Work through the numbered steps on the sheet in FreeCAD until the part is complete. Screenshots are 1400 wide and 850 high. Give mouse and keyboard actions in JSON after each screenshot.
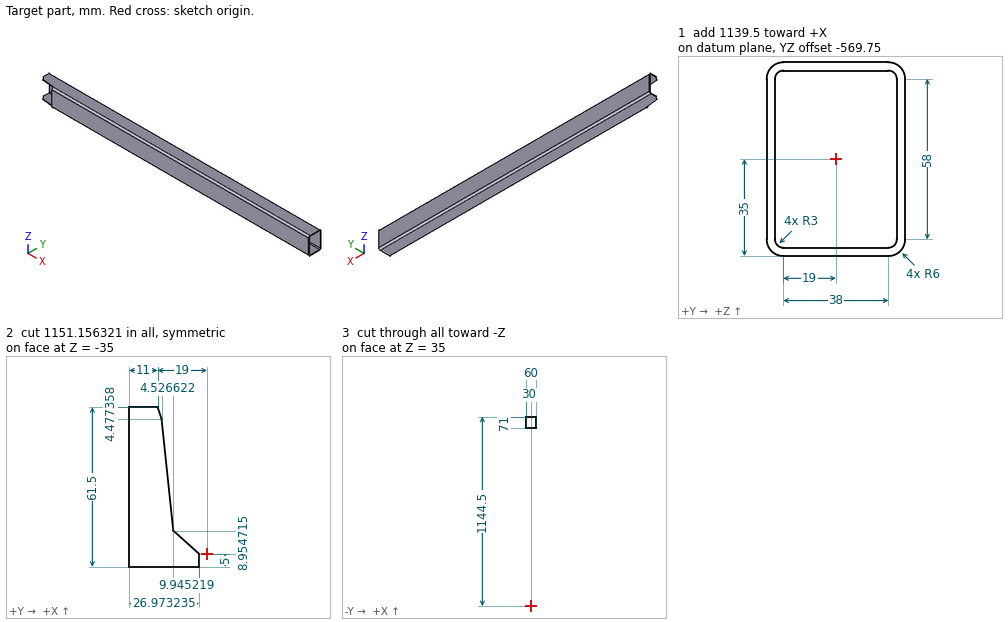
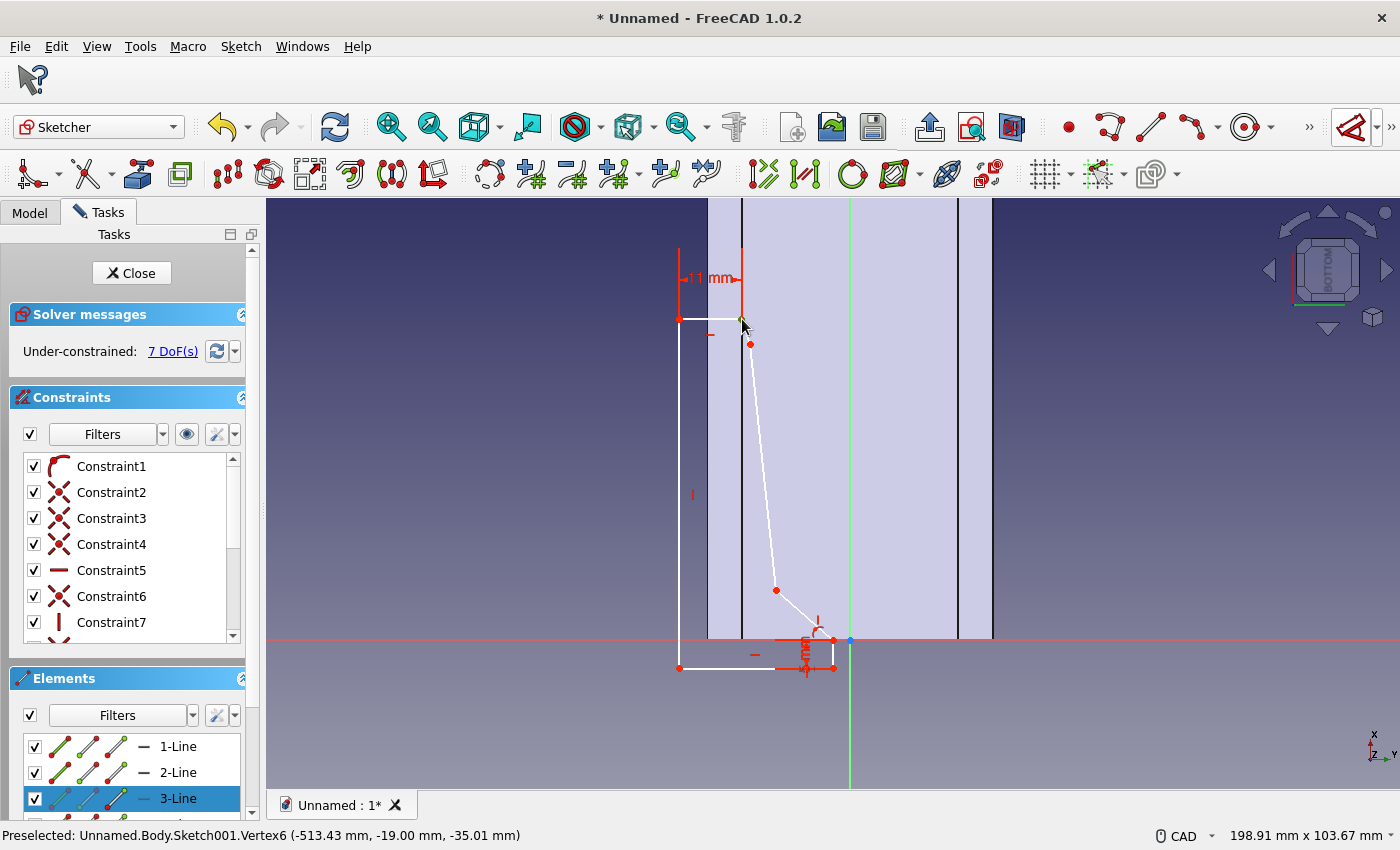
{"action": "left_click", "coordinate": [1376, 128]}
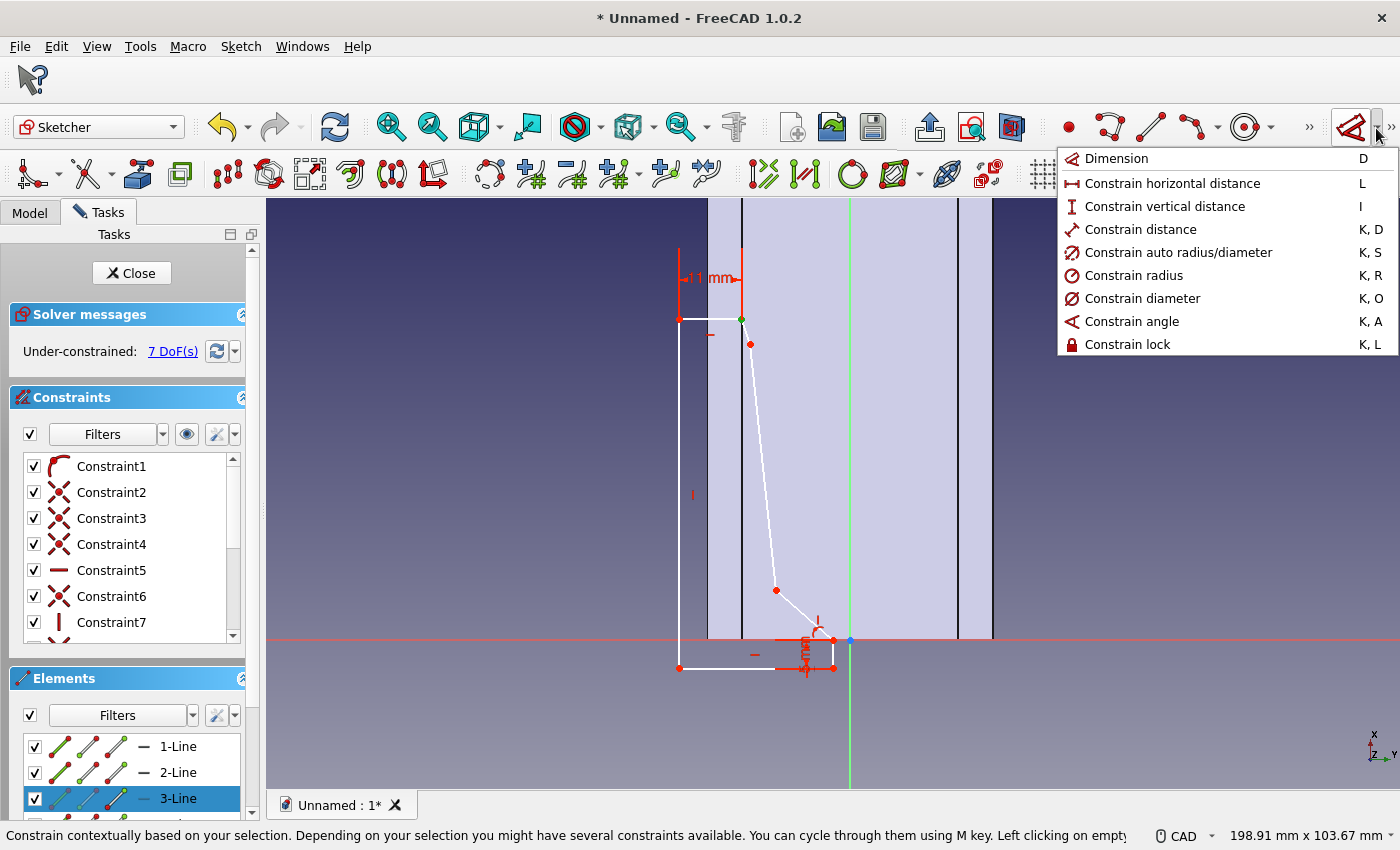
{"action": "left_click", "coordinate": [1228, 184]}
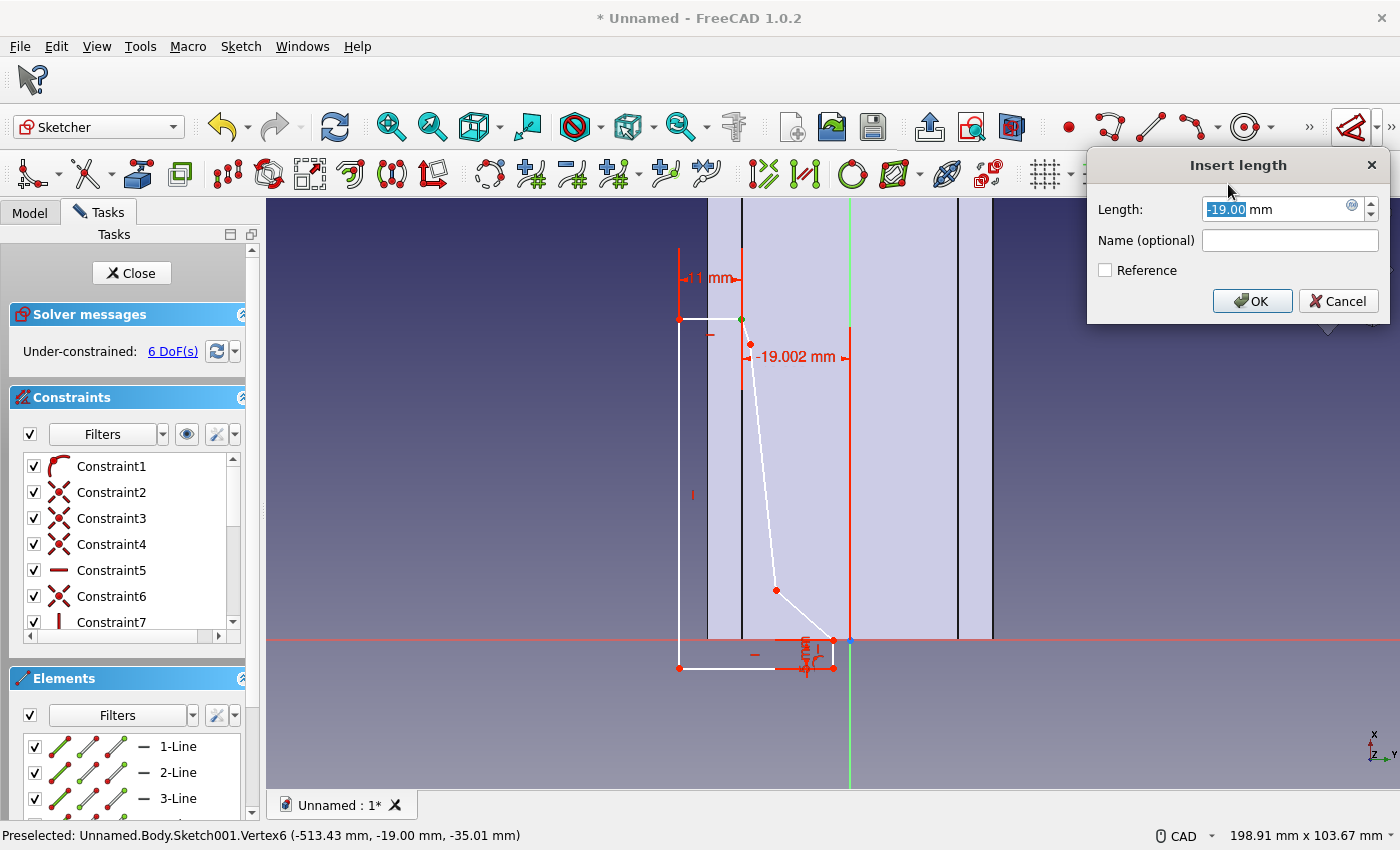
{"action": "type", "text": "-19"}
{"action": "key", "text": "Return"}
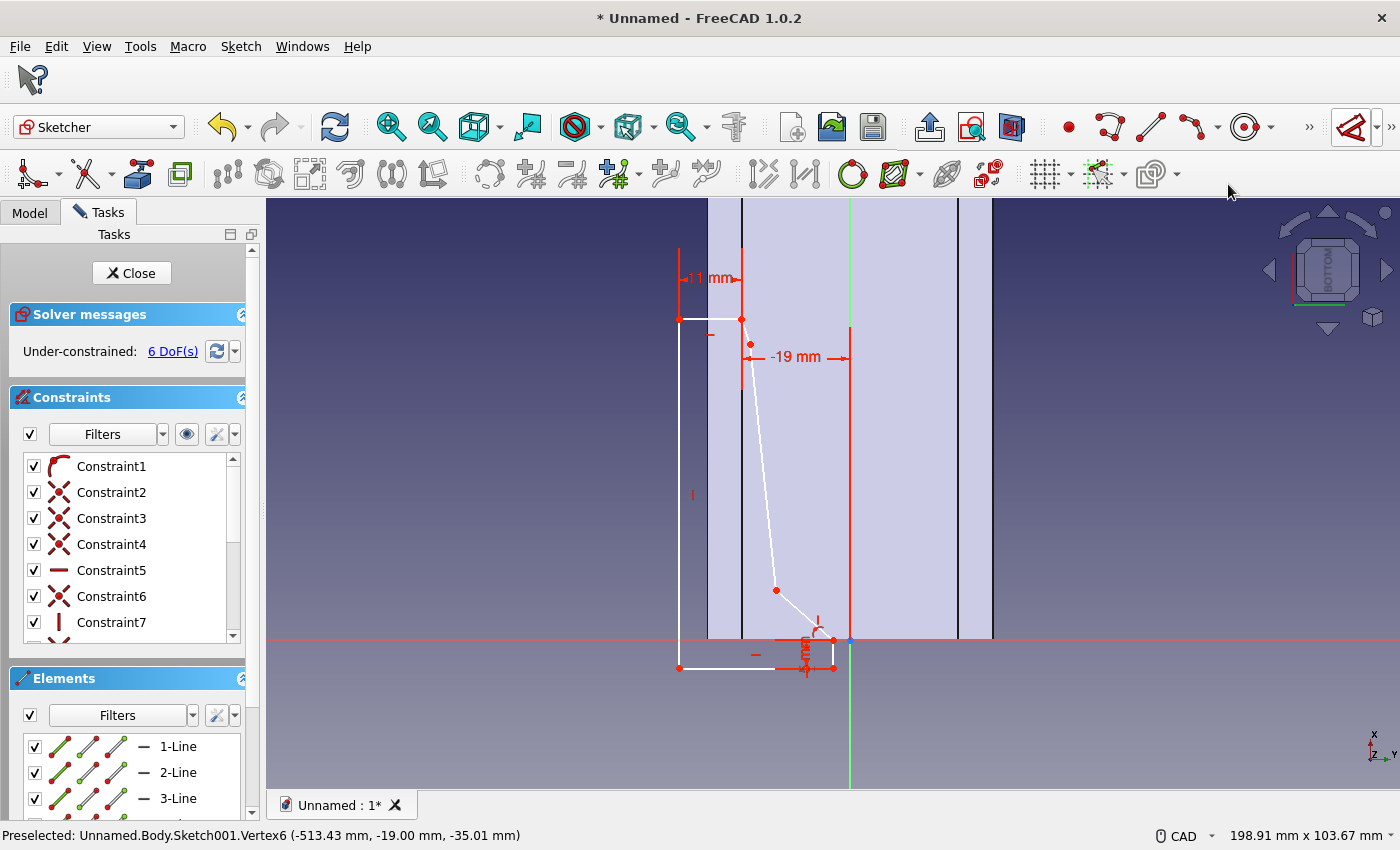
{"action": "left_click", "coordinate": [679, 424]}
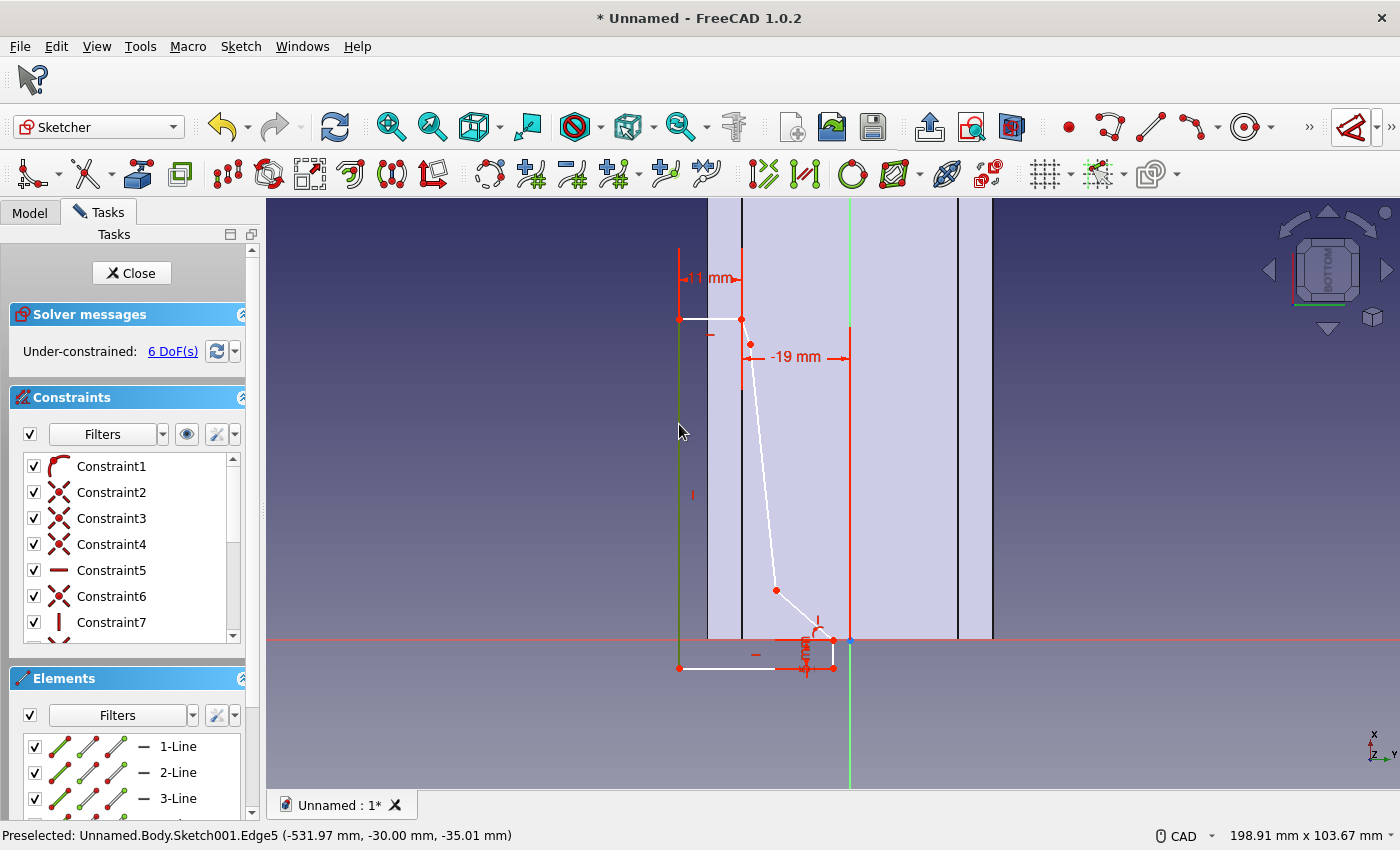
{"action": "key", "text": "i"}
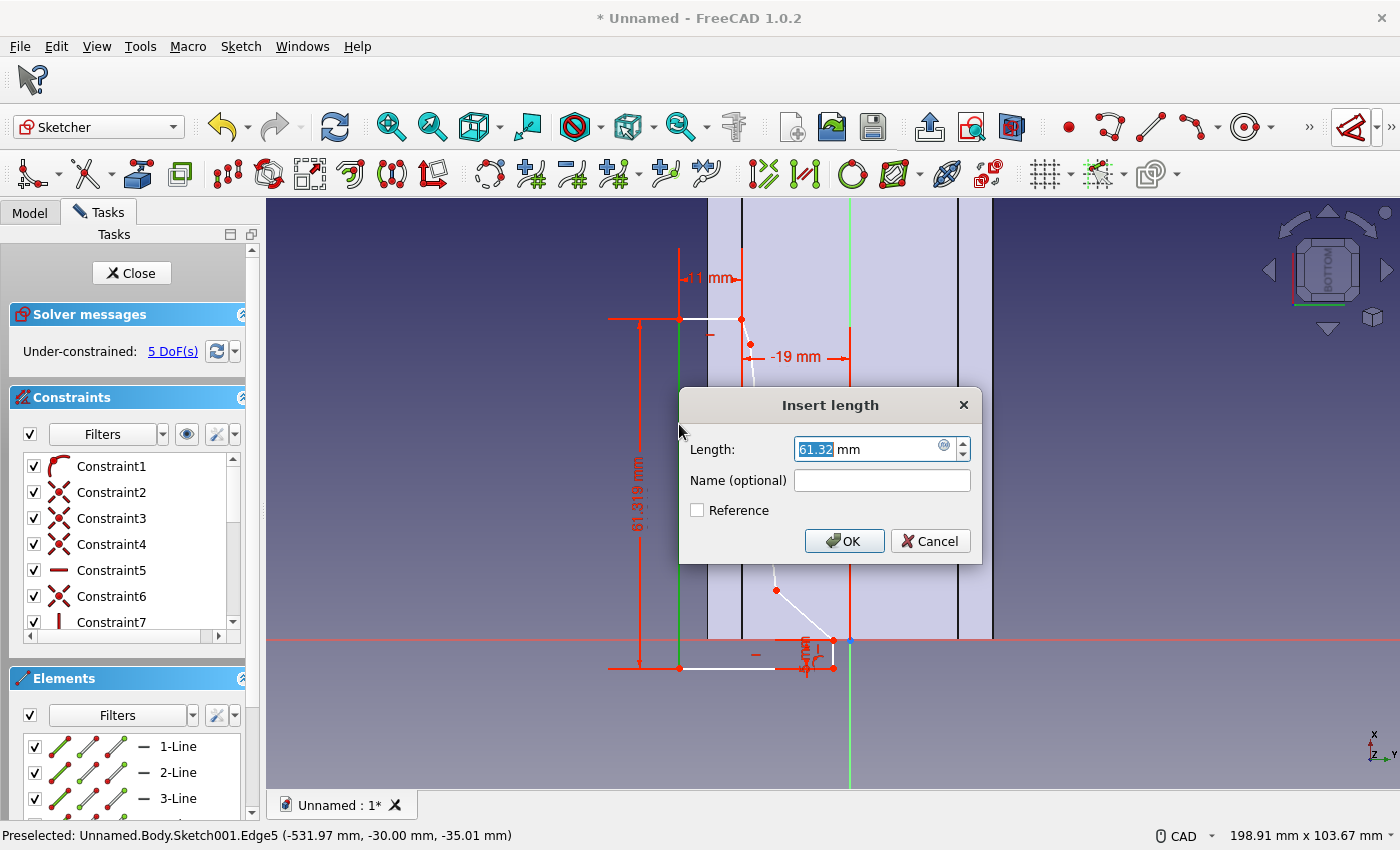
{"action": "type", "text": "61.5"}
{"action": "key", "text": "Return"}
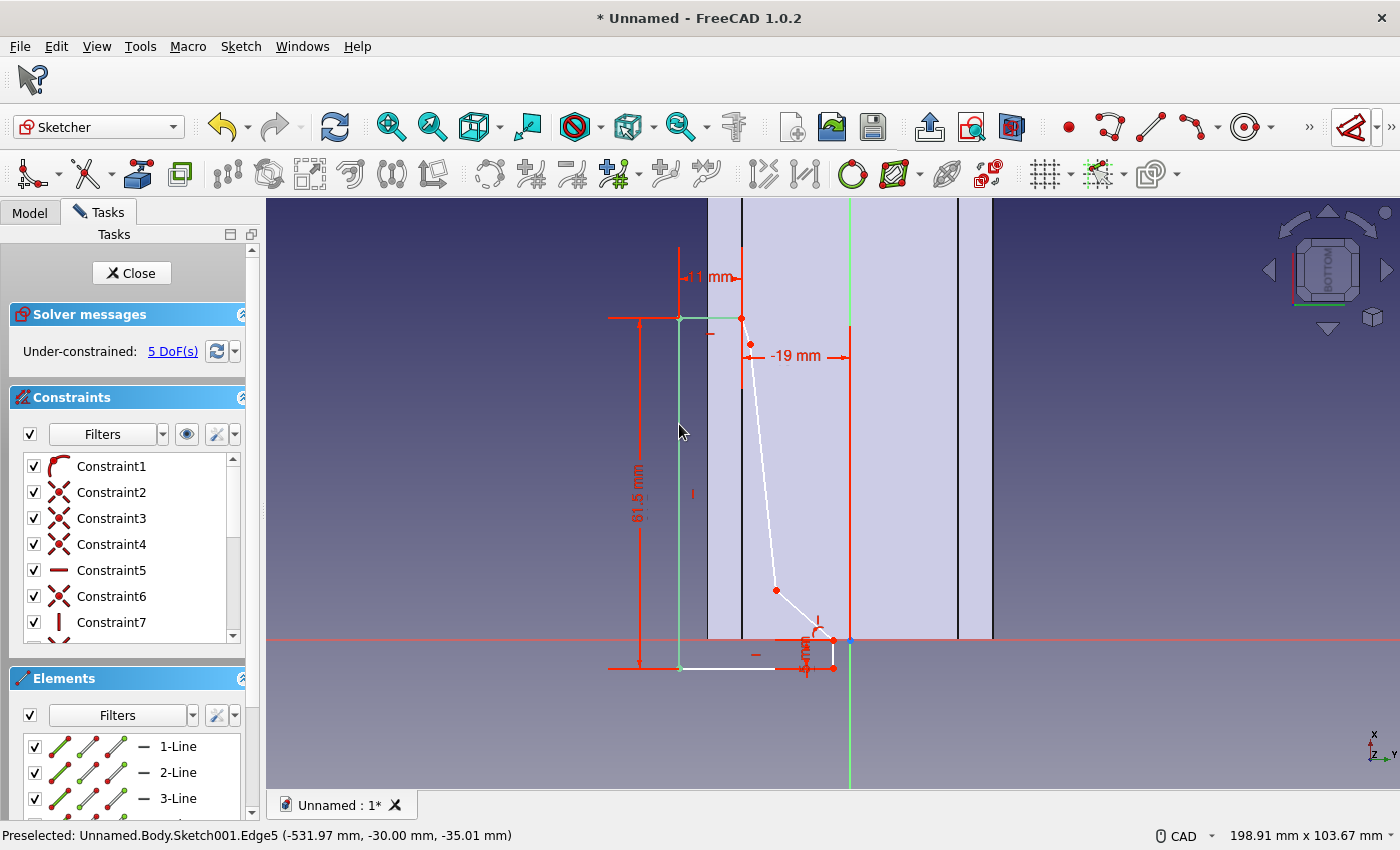
{"action": "left_click", "coordinate": [725, 669]}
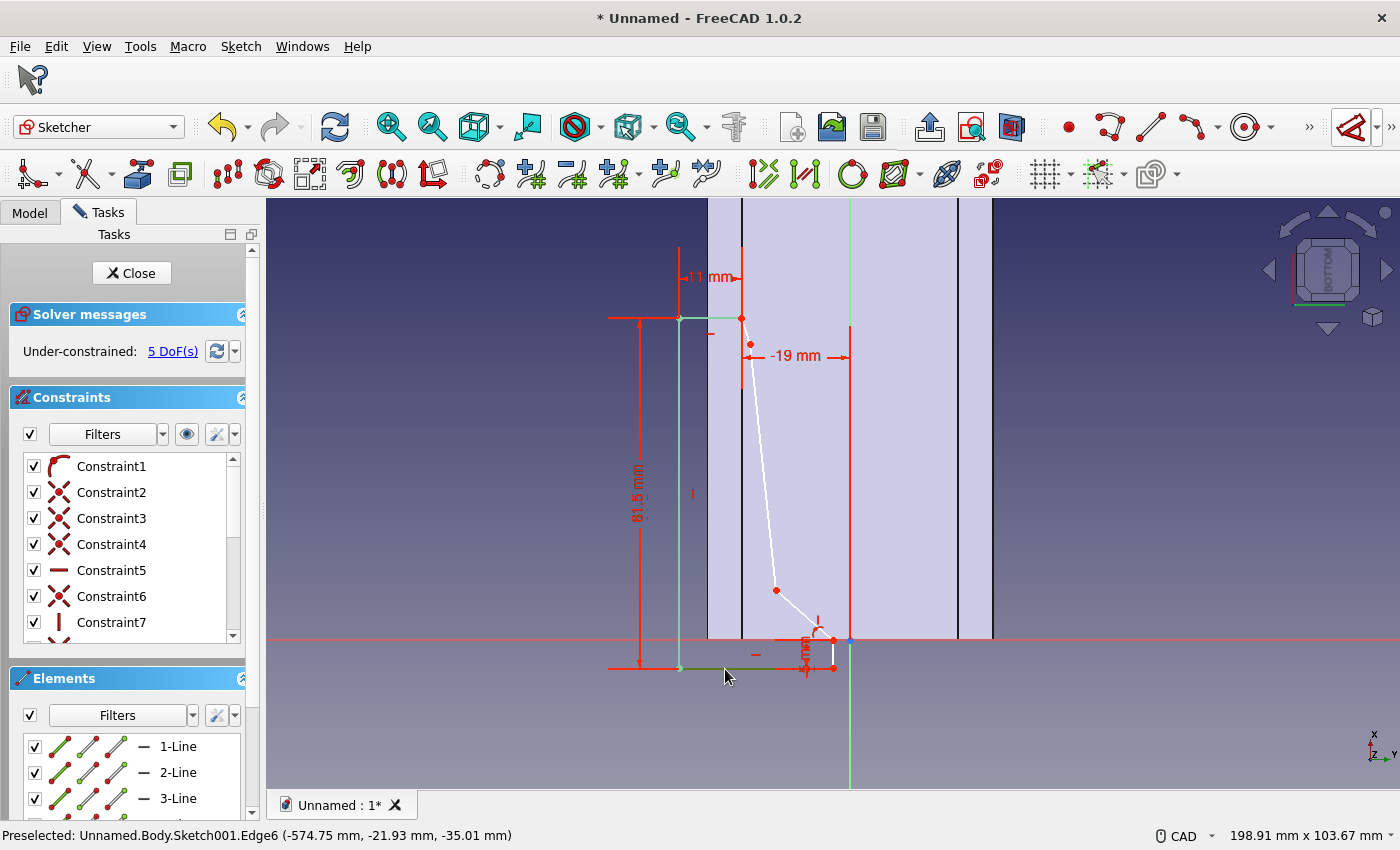
{"action": "key", "text": "l"}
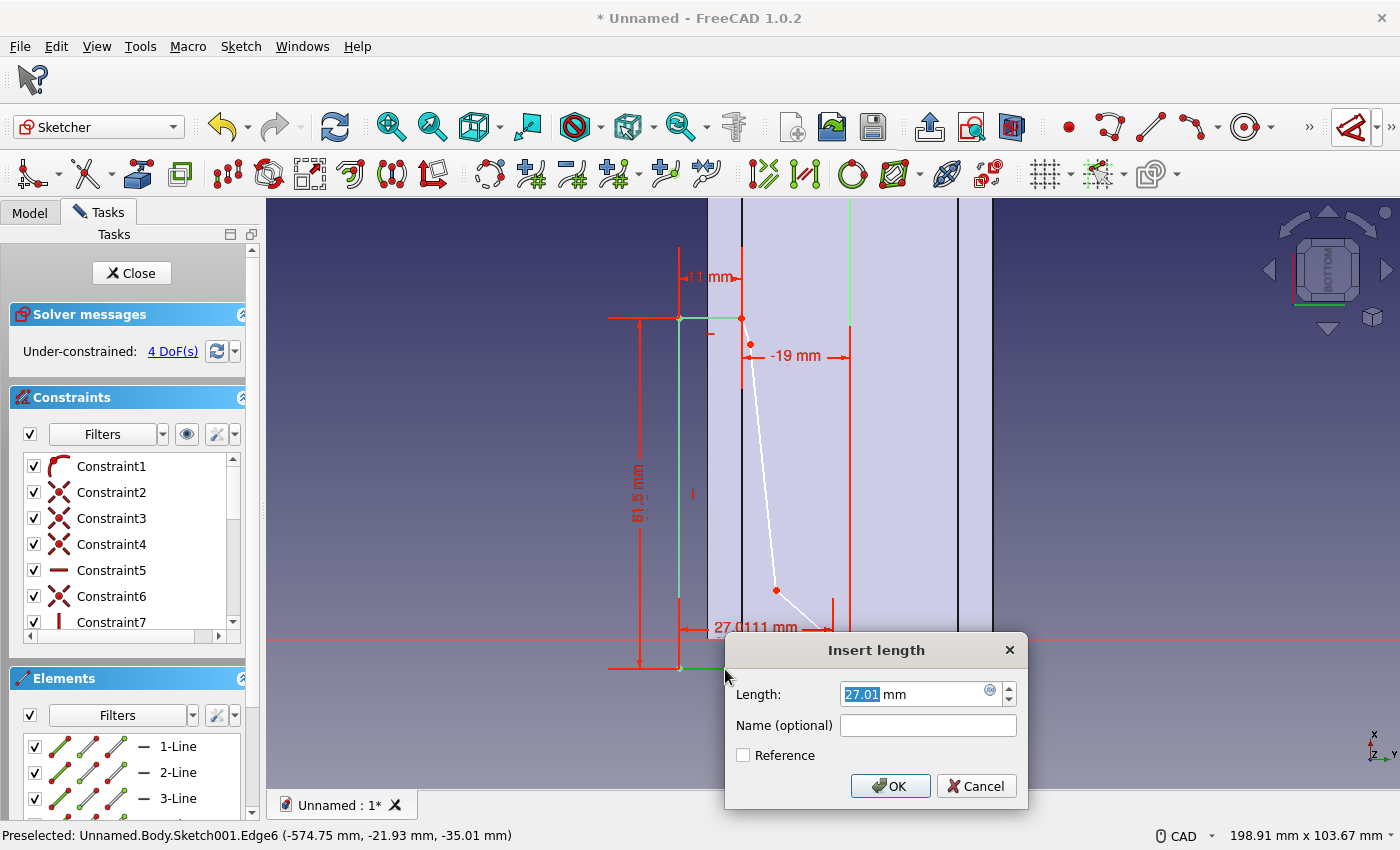
{"action": "type", "text": "26.973235"}
{"action": "key", "text": "Return"}